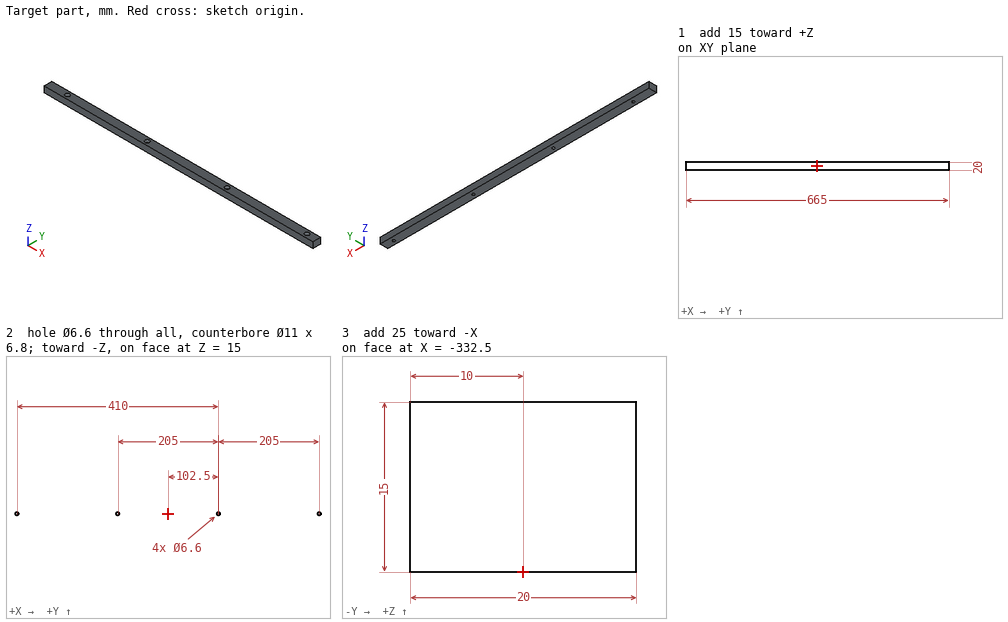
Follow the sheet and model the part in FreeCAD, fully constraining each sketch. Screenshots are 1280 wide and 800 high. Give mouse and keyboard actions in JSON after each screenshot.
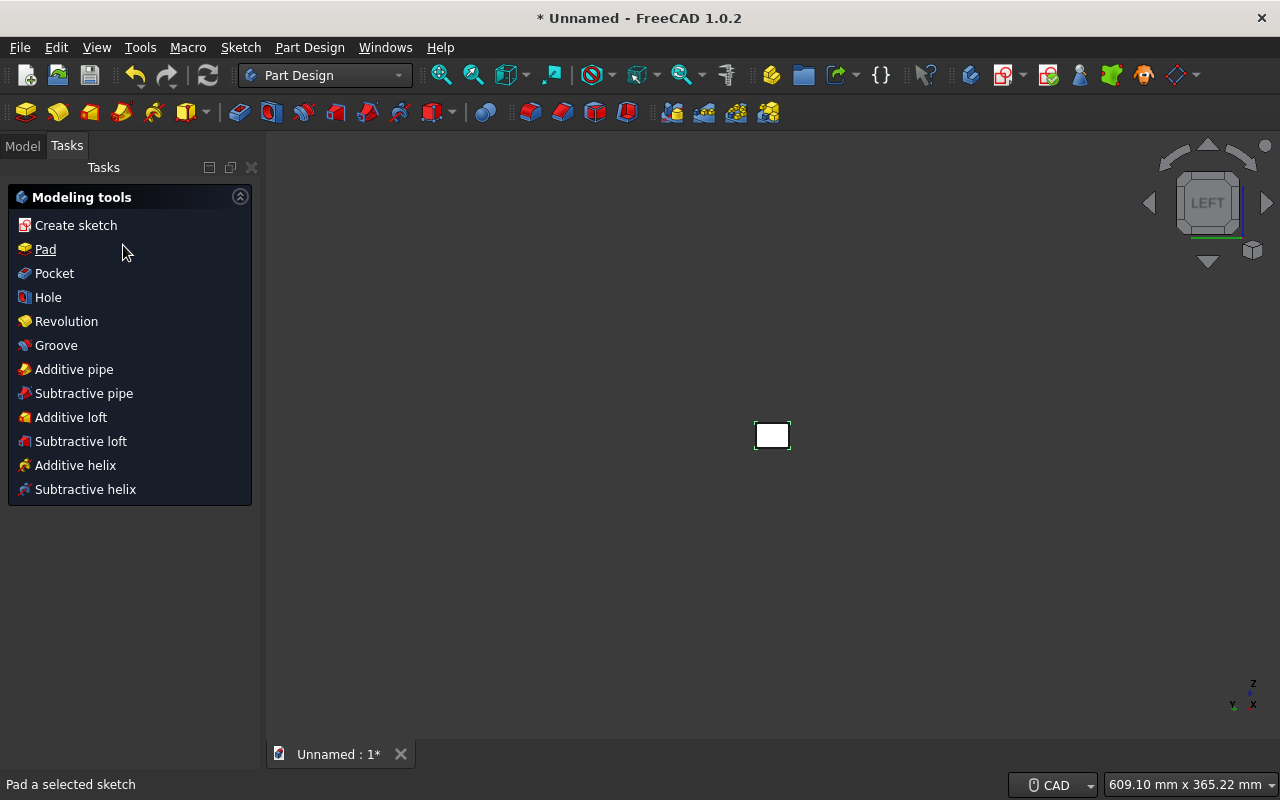
{"action": "left_click", "coordinate": [26, 112]}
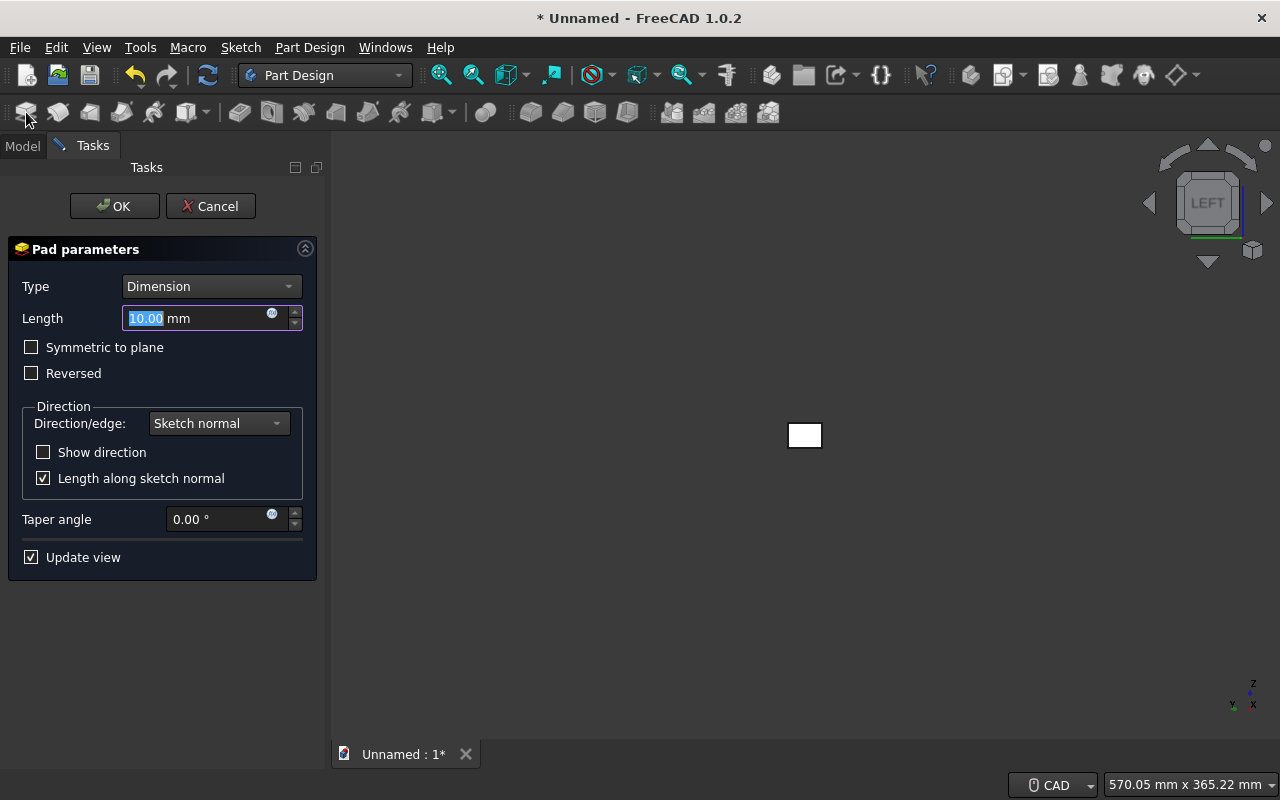
{"action": "type", "text": "25"}
{"action": "key", "text": "Tab"}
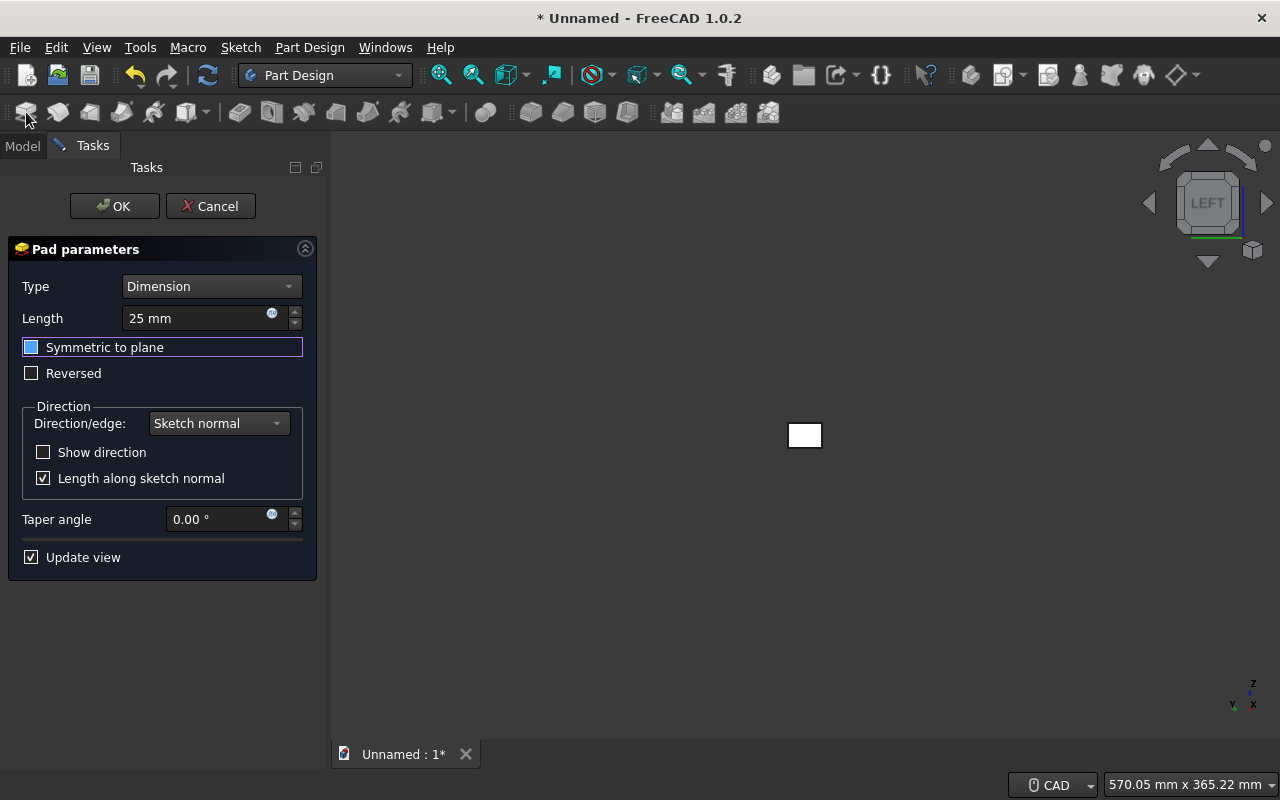
{"action": "left_click", "coordinate": [115, 206]}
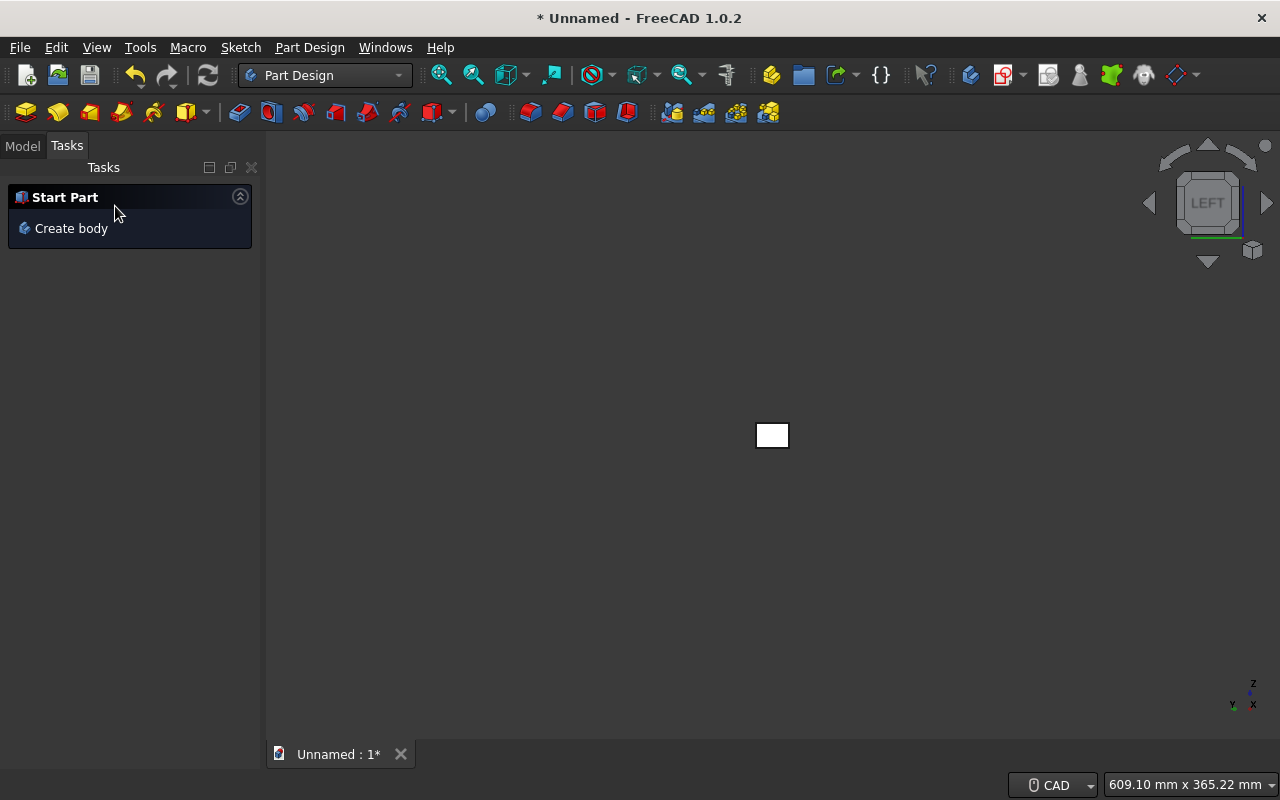
{"action": "key", "text": "0"}